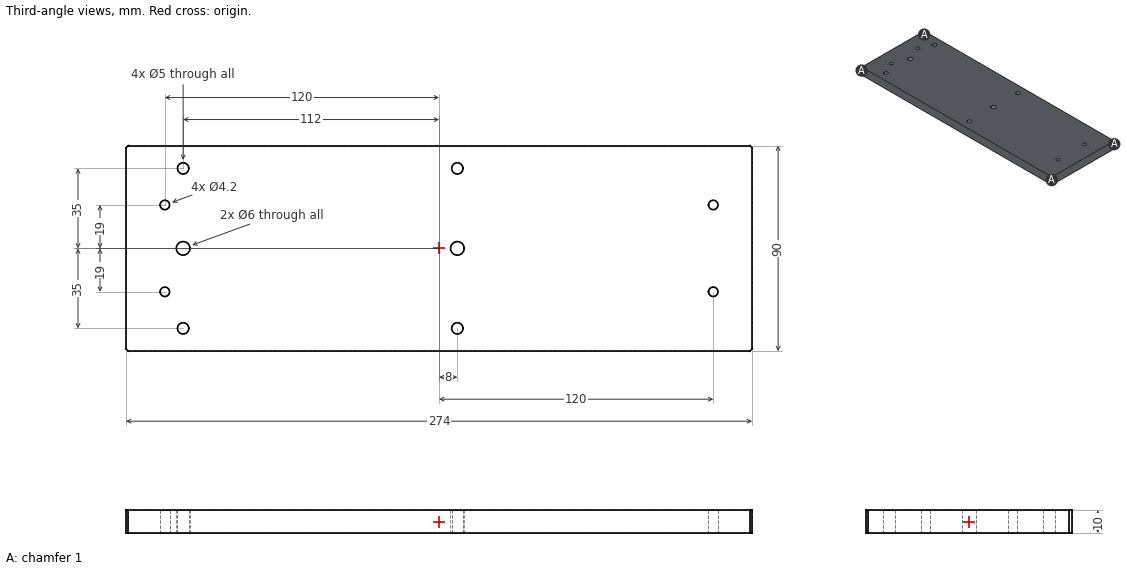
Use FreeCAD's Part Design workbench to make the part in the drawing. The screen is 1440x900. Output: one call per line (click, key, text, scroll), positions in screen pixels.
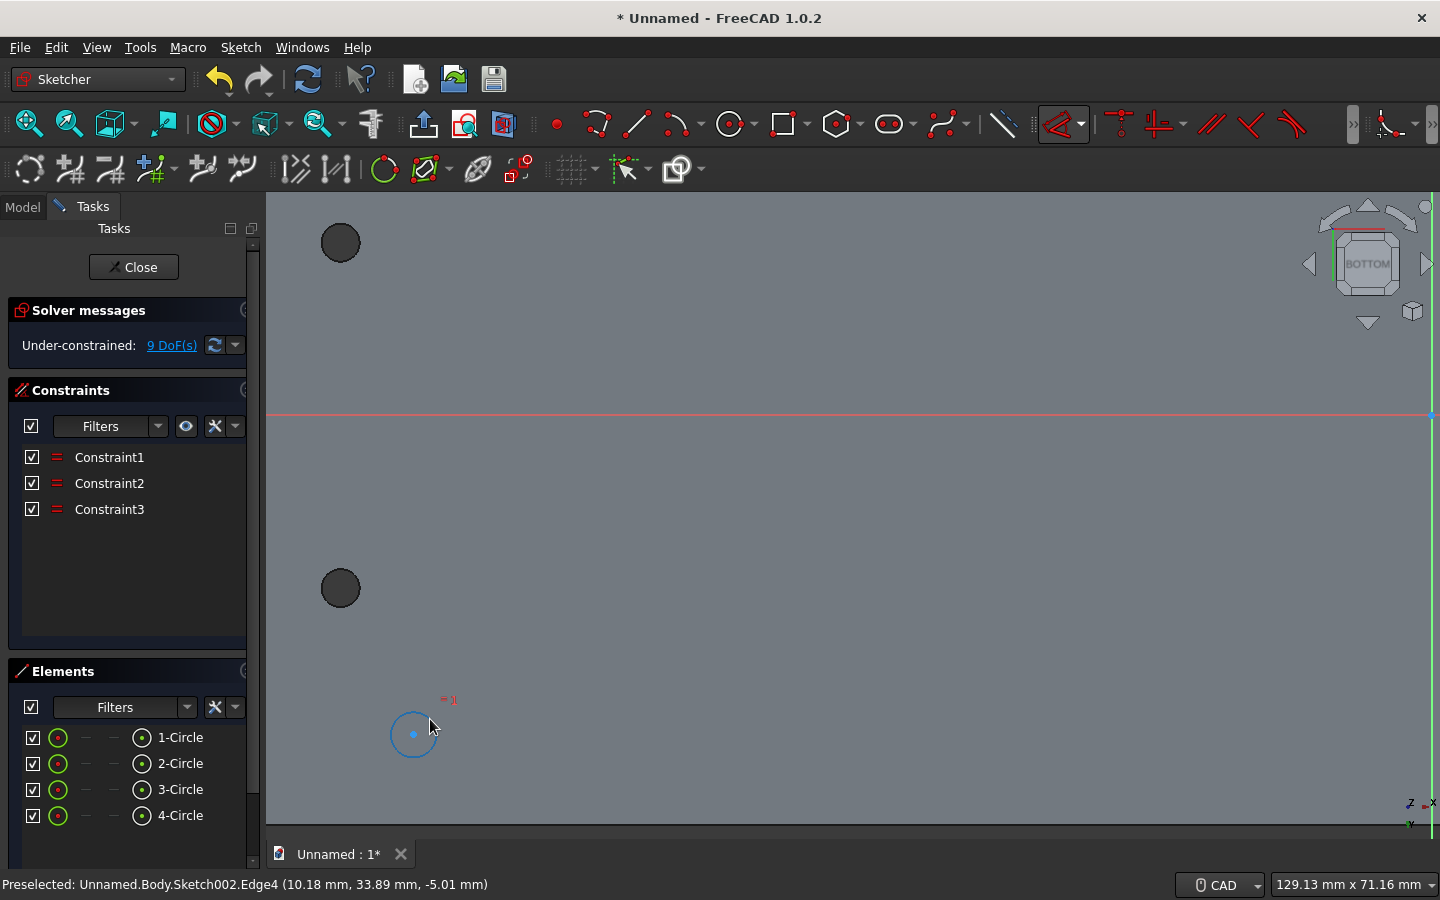
click(430, 719)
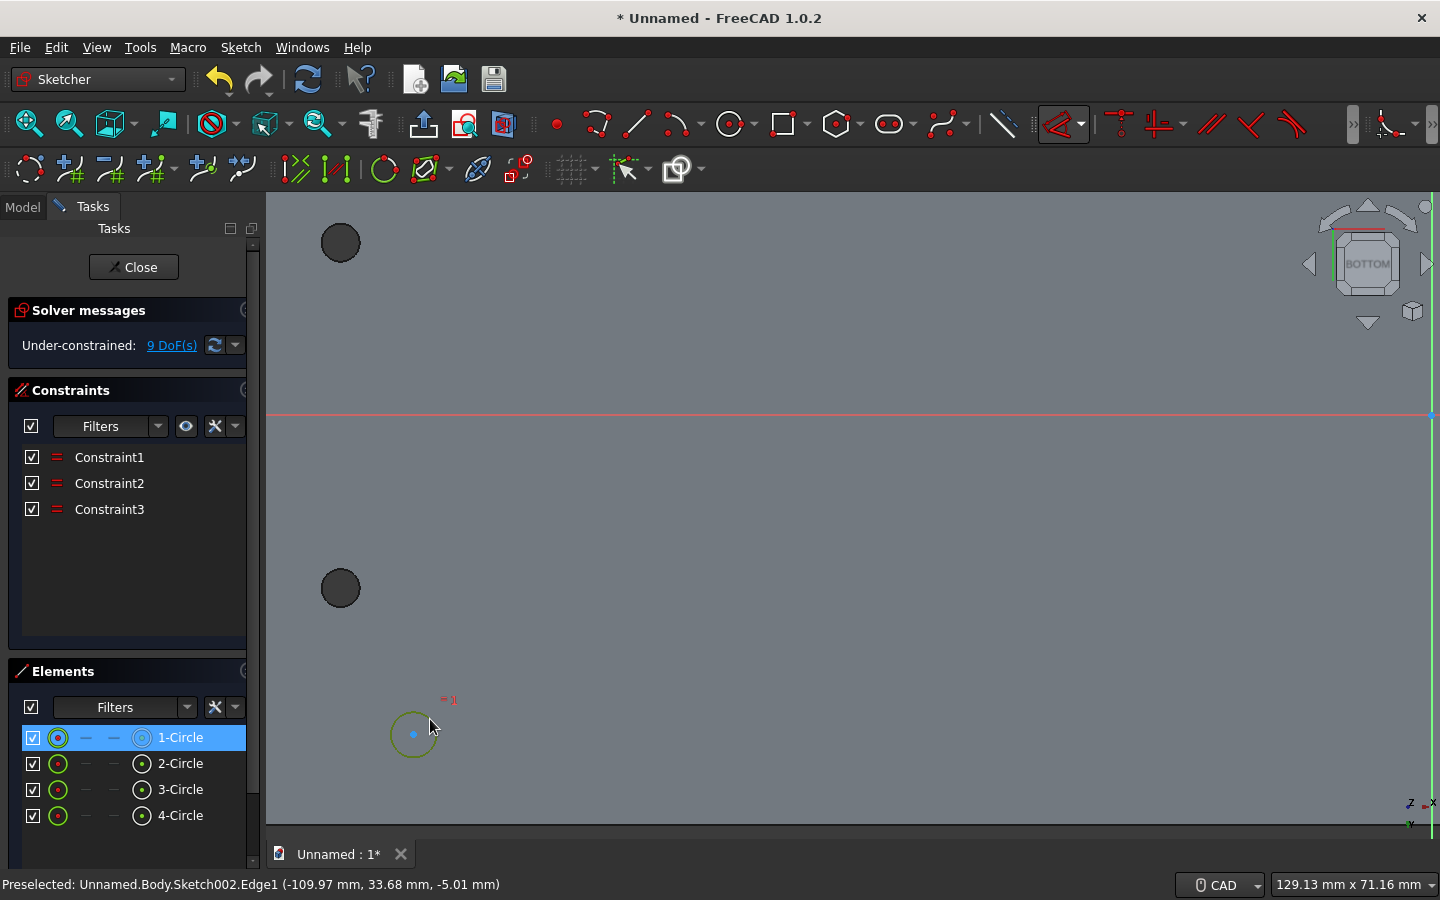
key(k)
key(o)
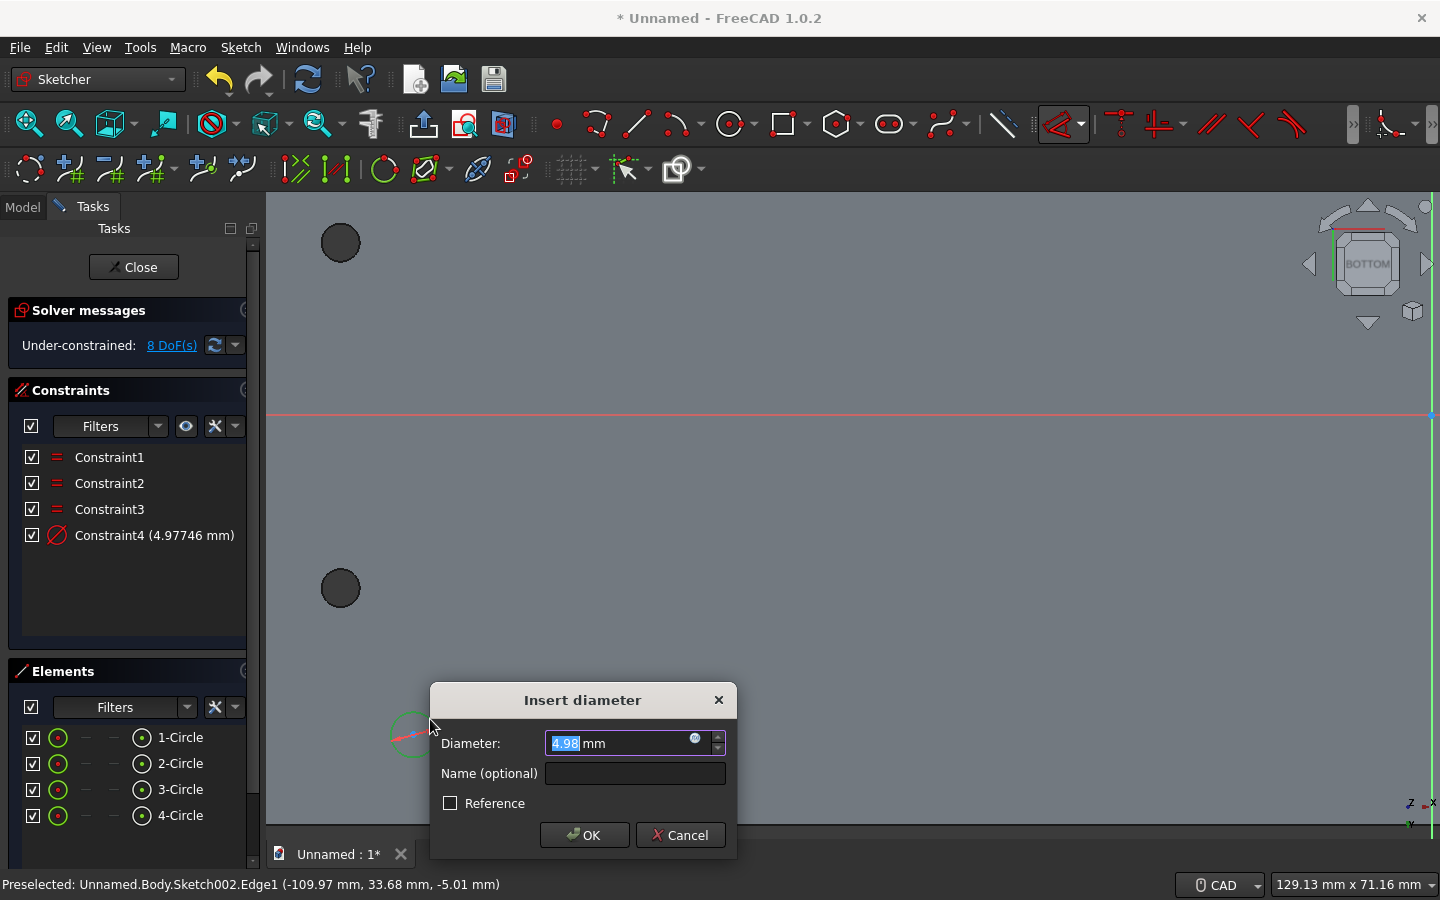
text(5)
key(Return)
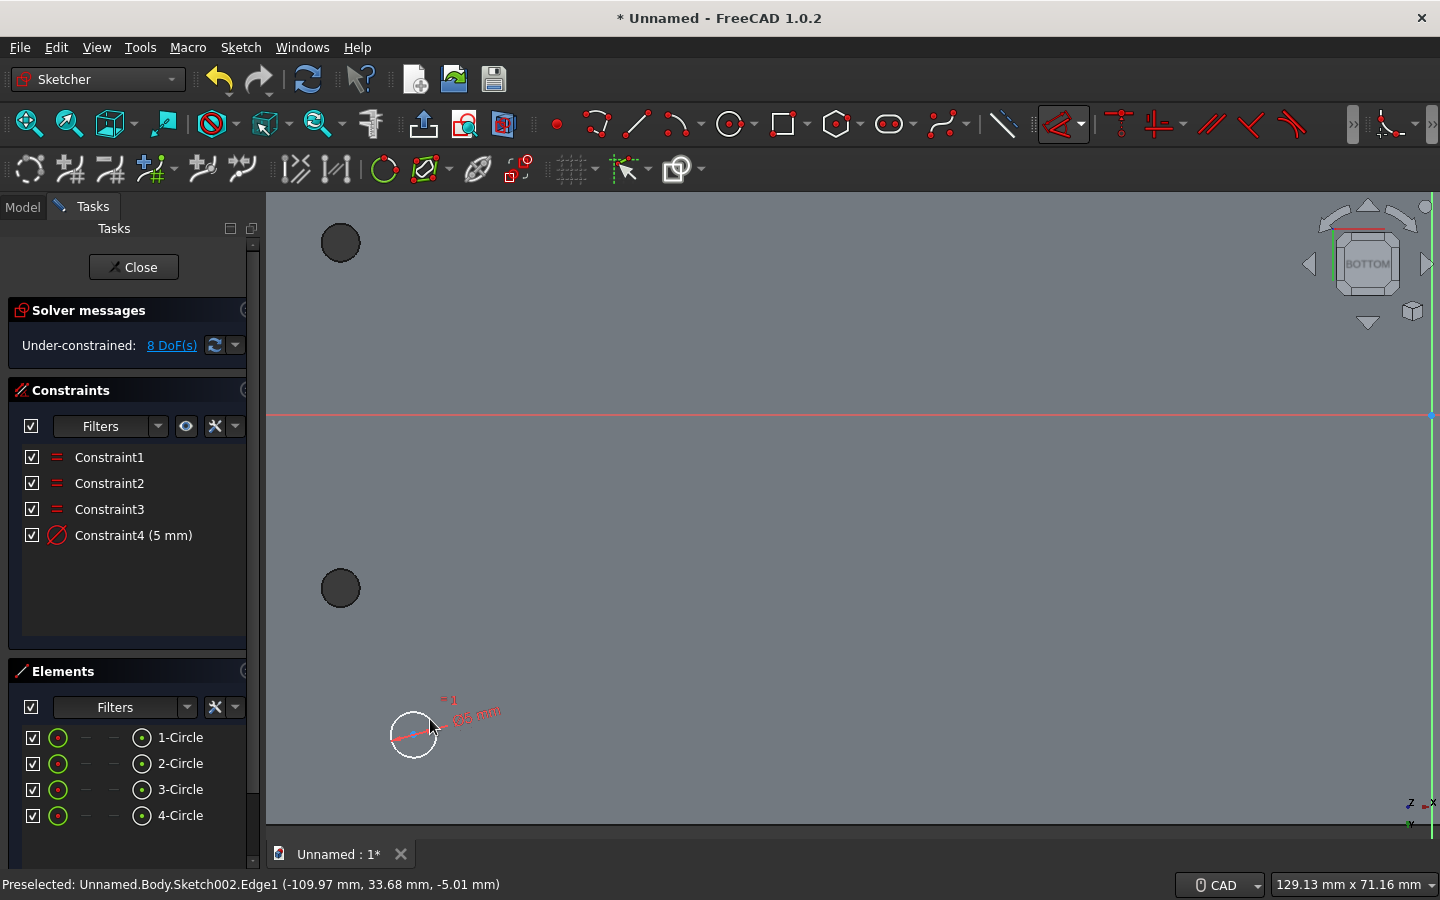
scroll(430, 719, down, 2)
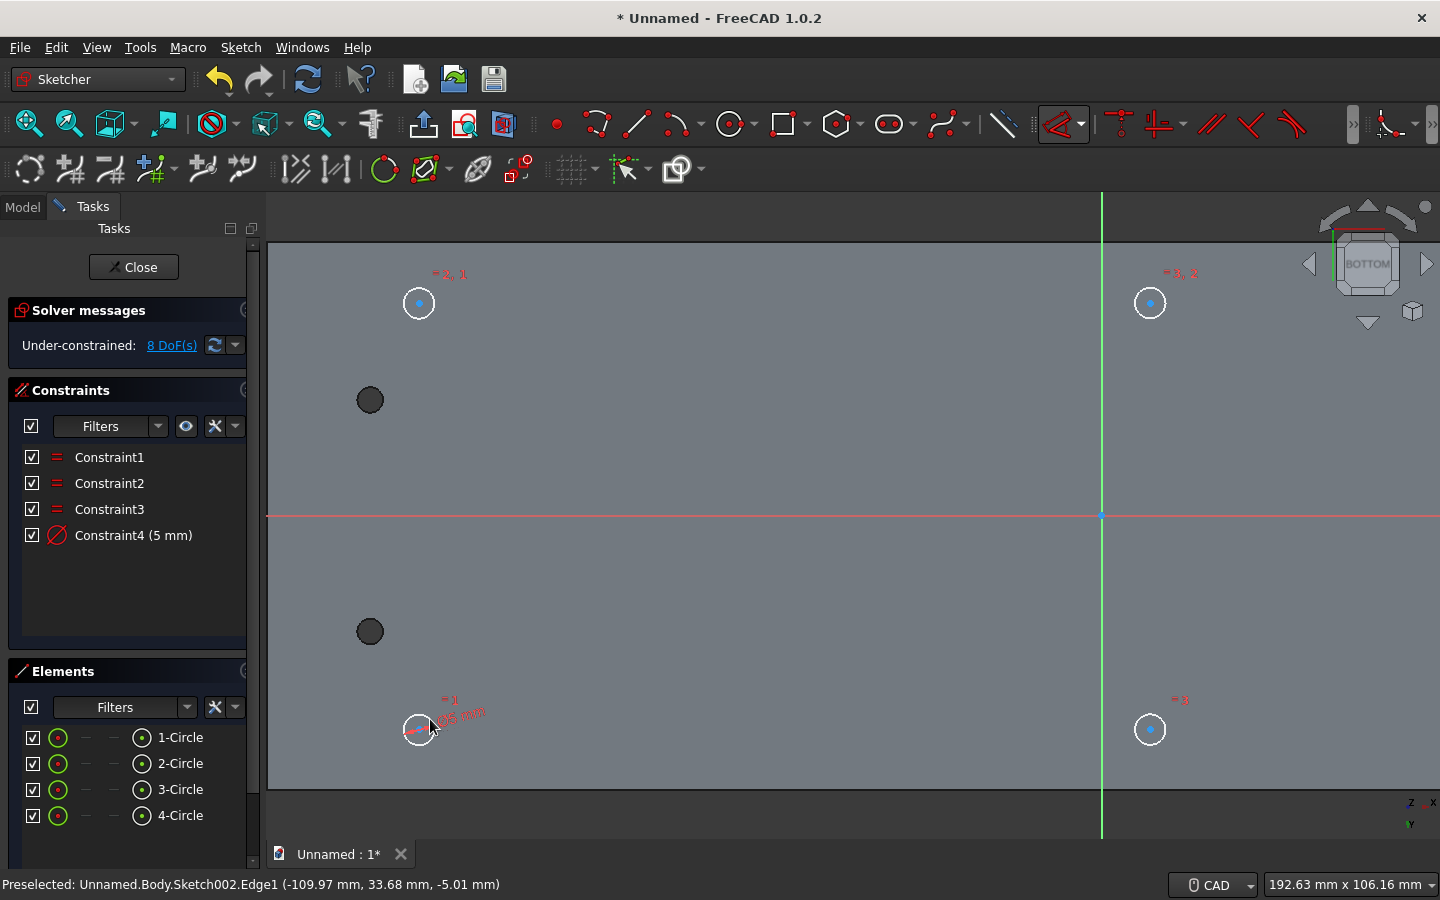
click(1150, 303)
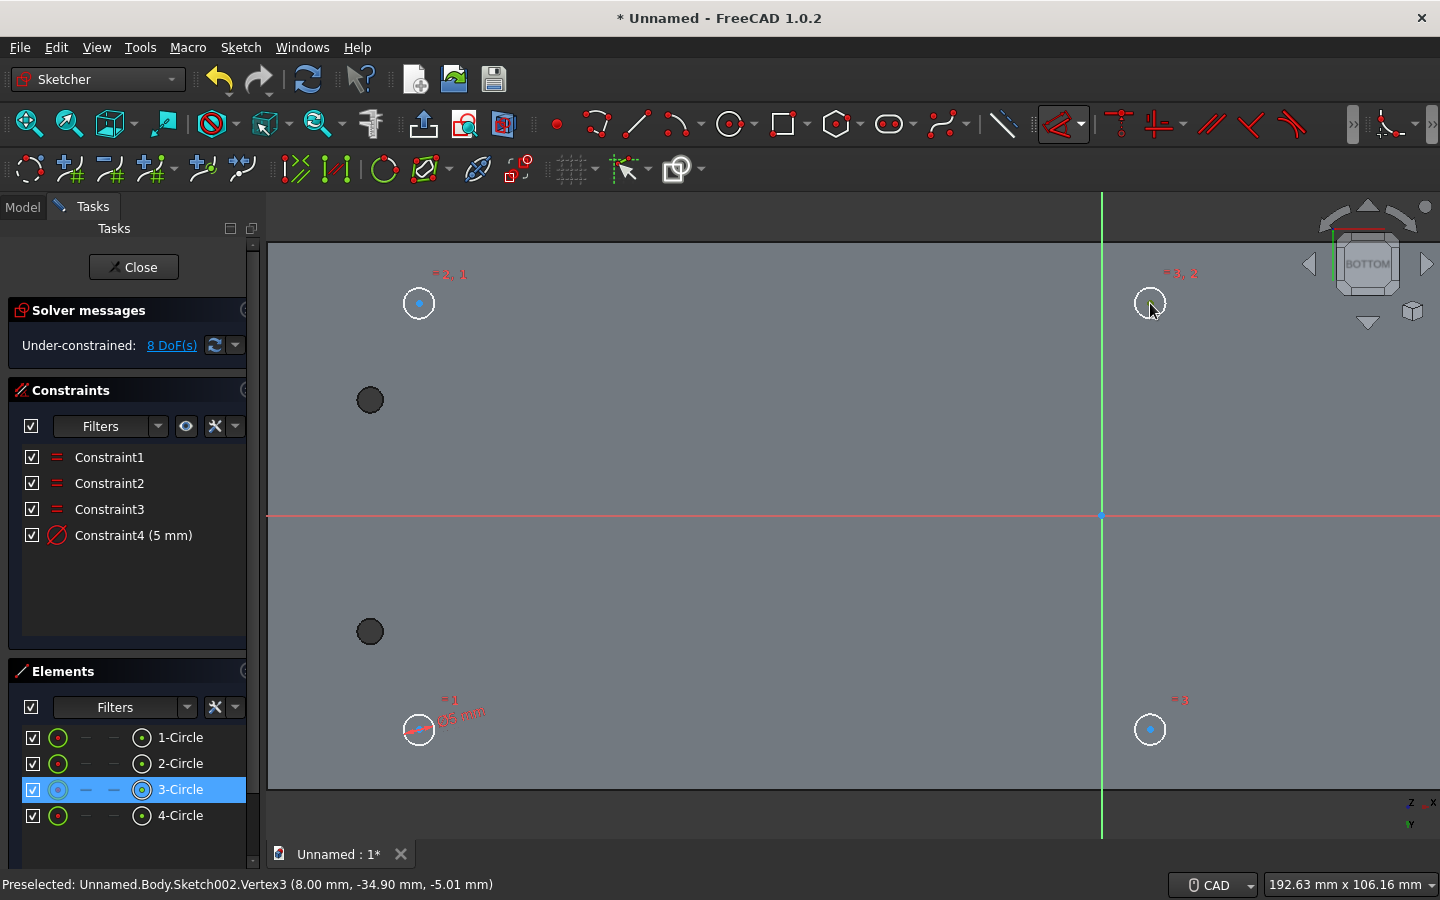
click(1084, 124)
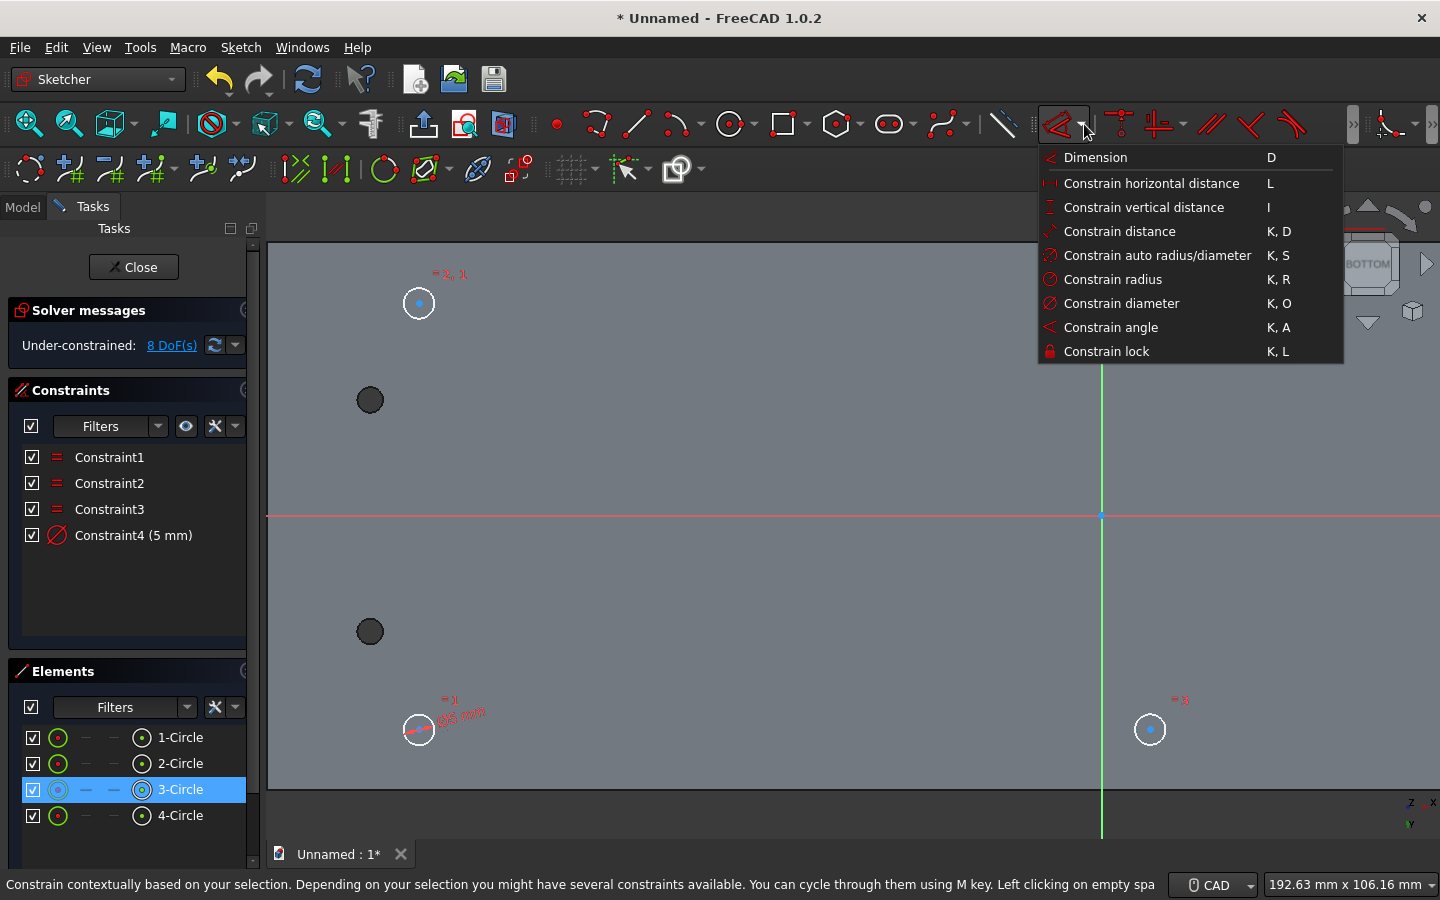
click(1191, 183)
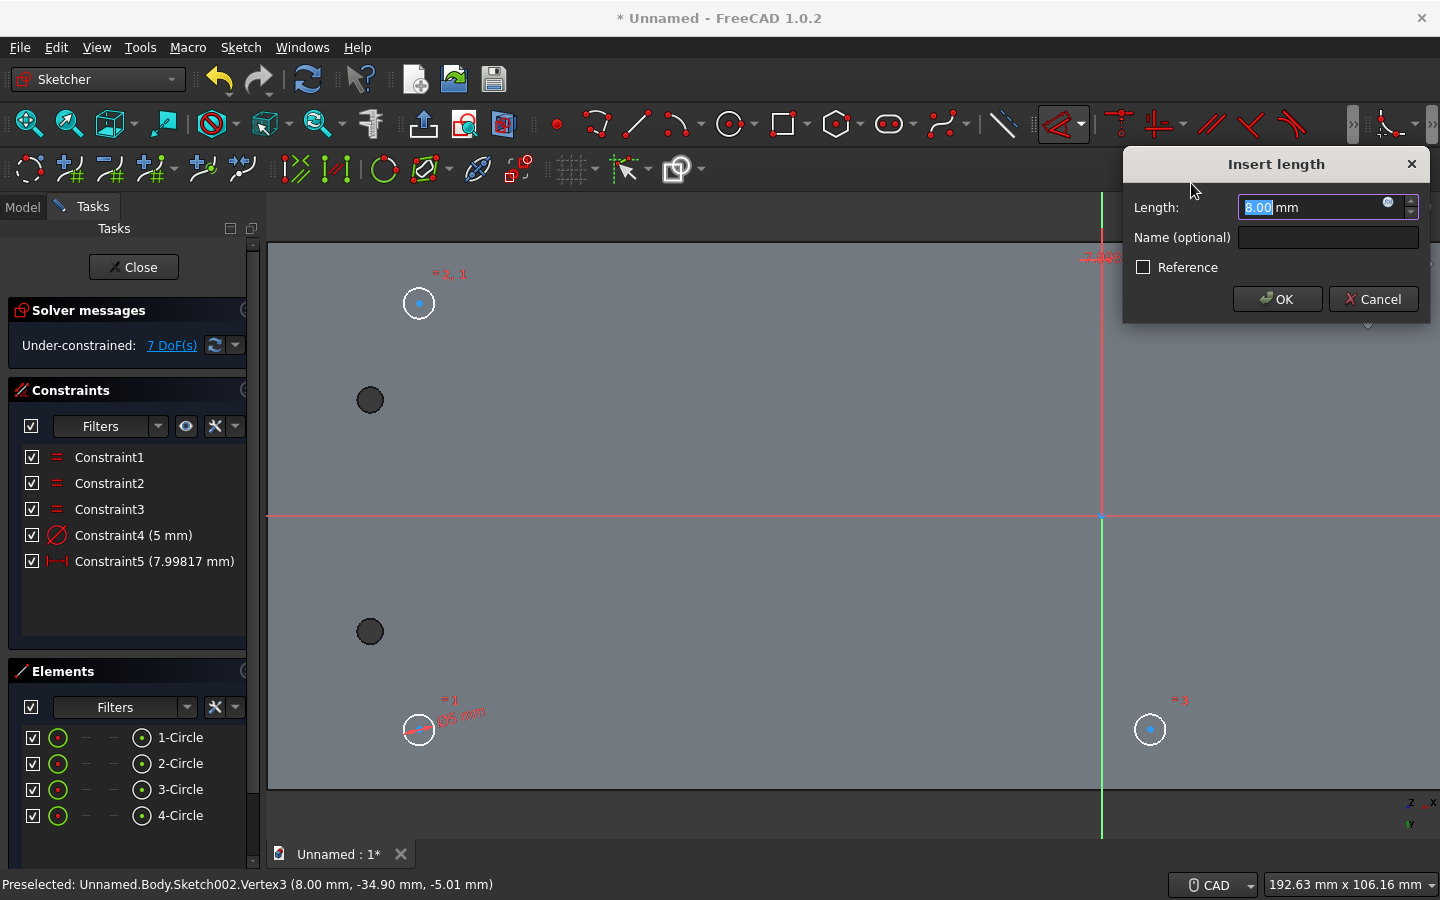
text(8)
key(Return)